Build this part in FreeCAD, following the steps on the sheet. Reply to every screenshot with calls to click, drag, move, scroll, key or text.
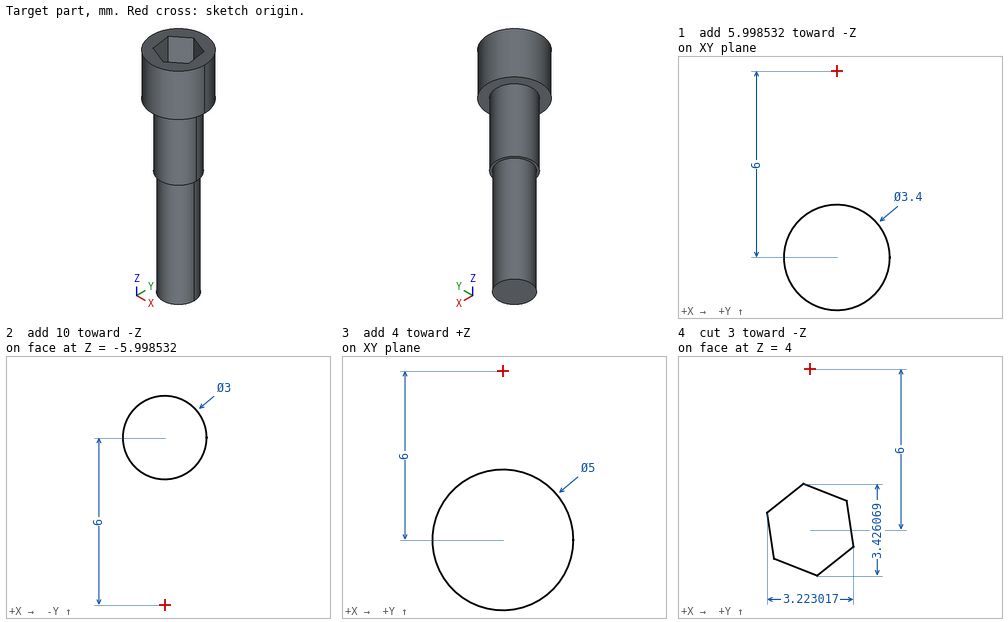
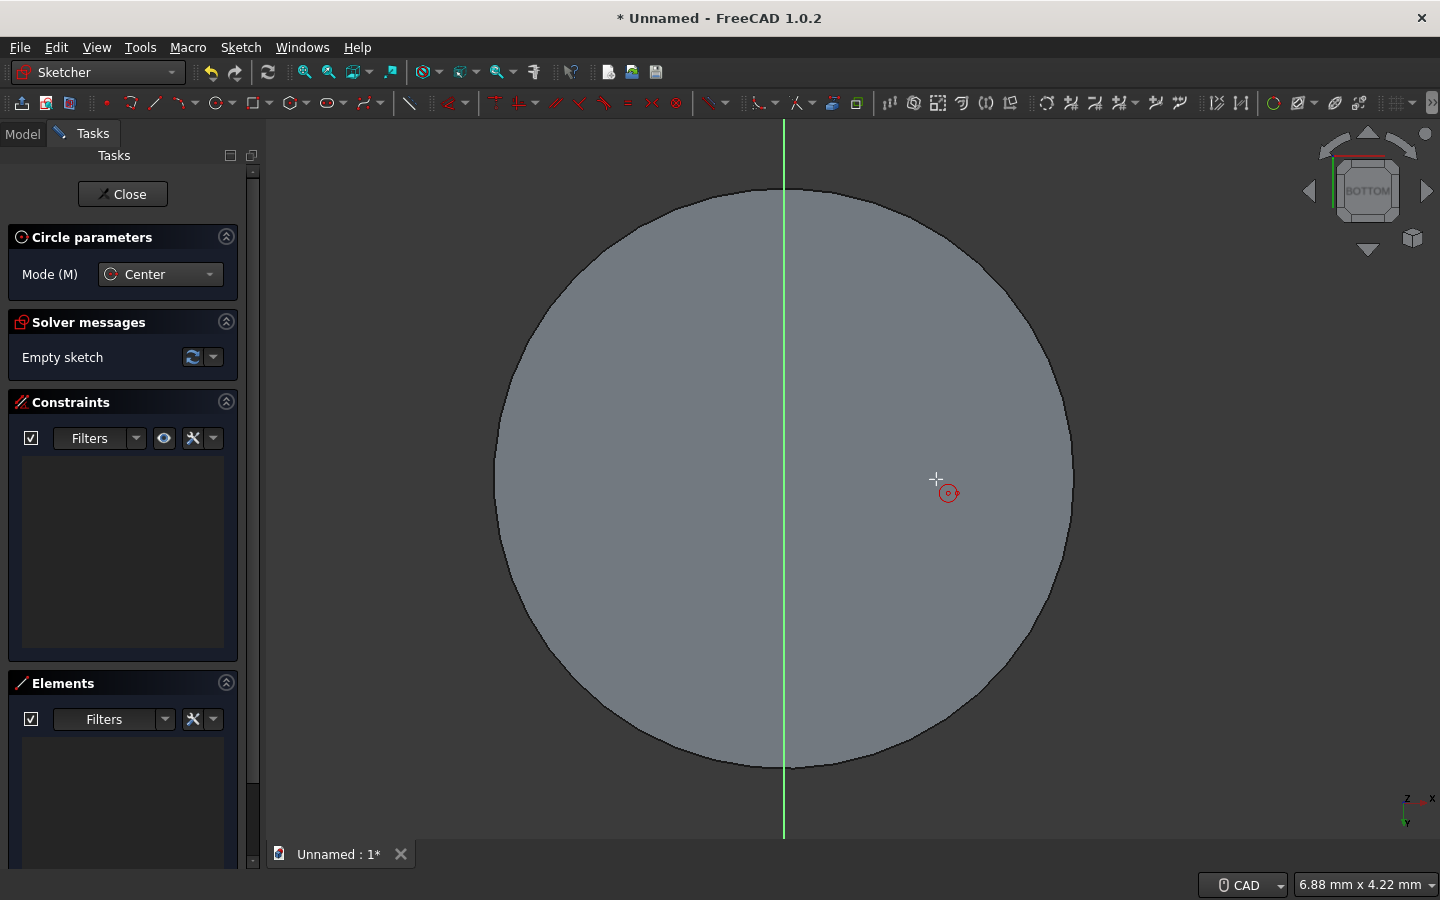
click(784, 479)
click(965, 298)
key(Escape)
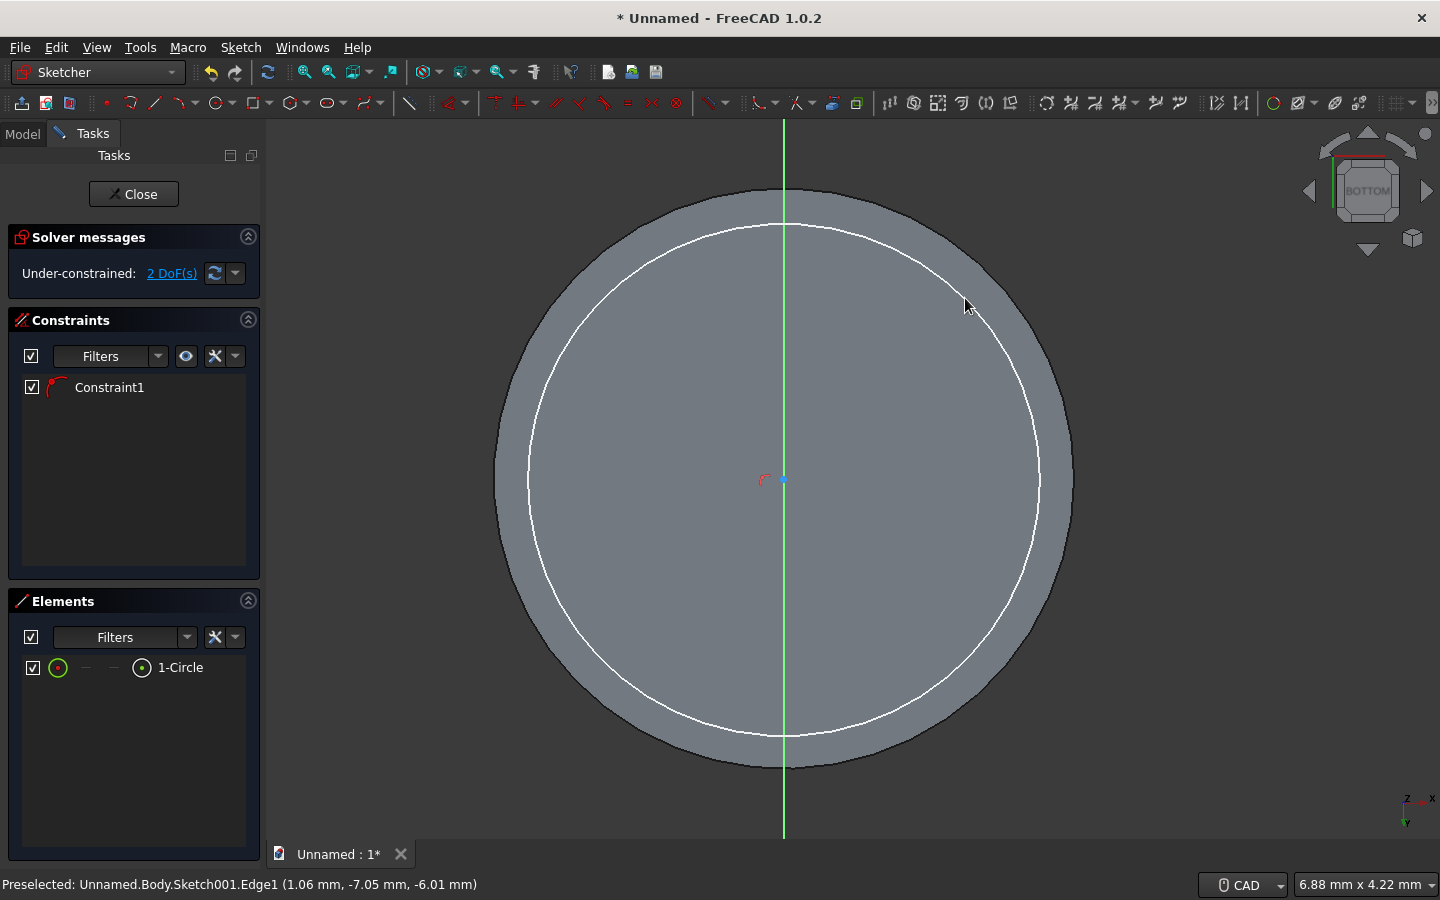
key(d)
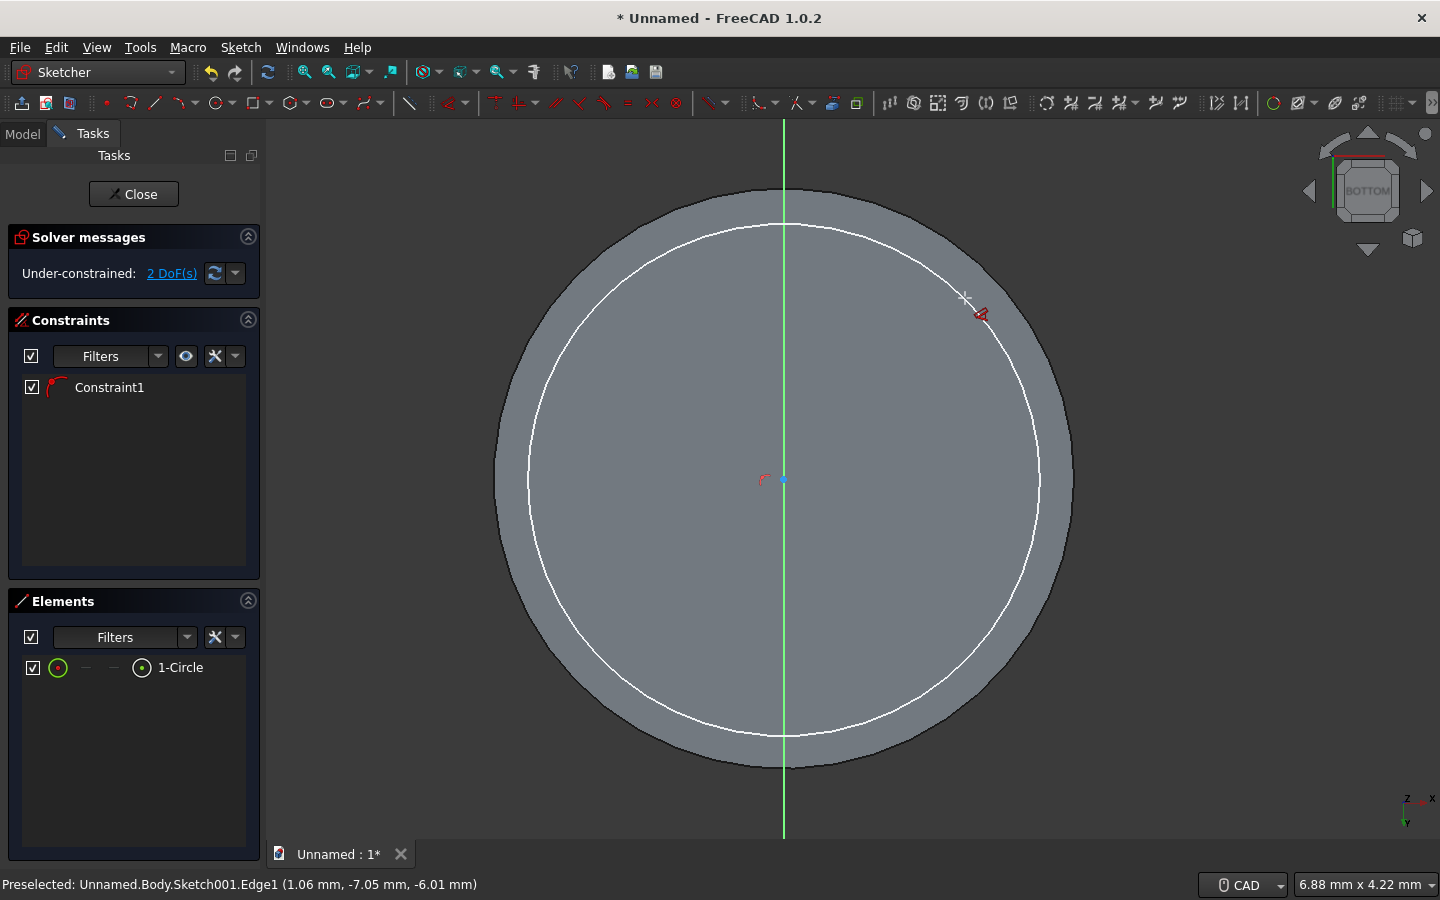
click(964, 298)
click(987, 275)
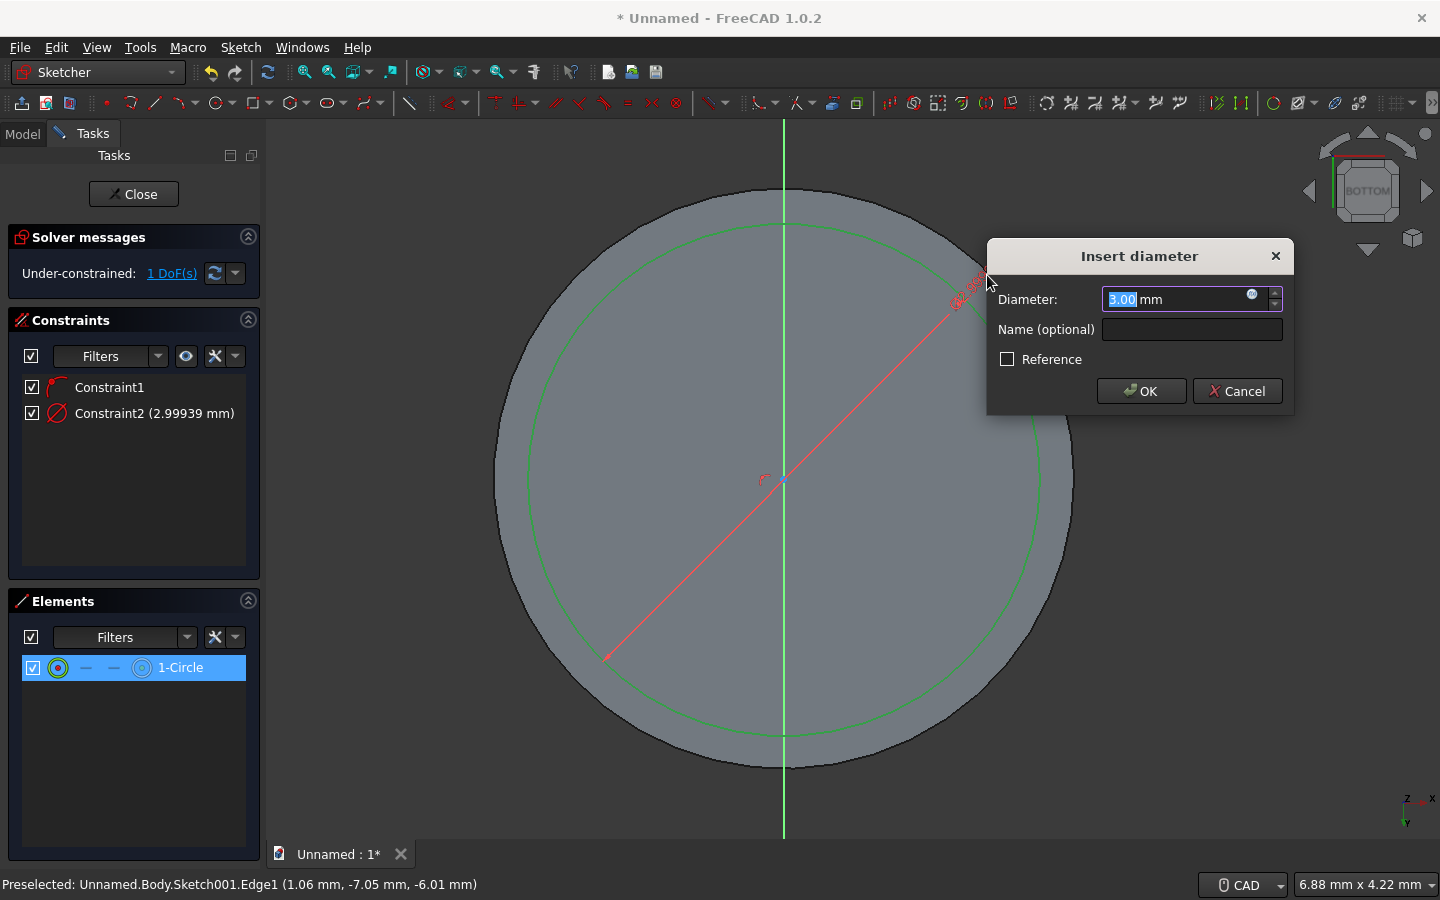
text(3)
key(Return)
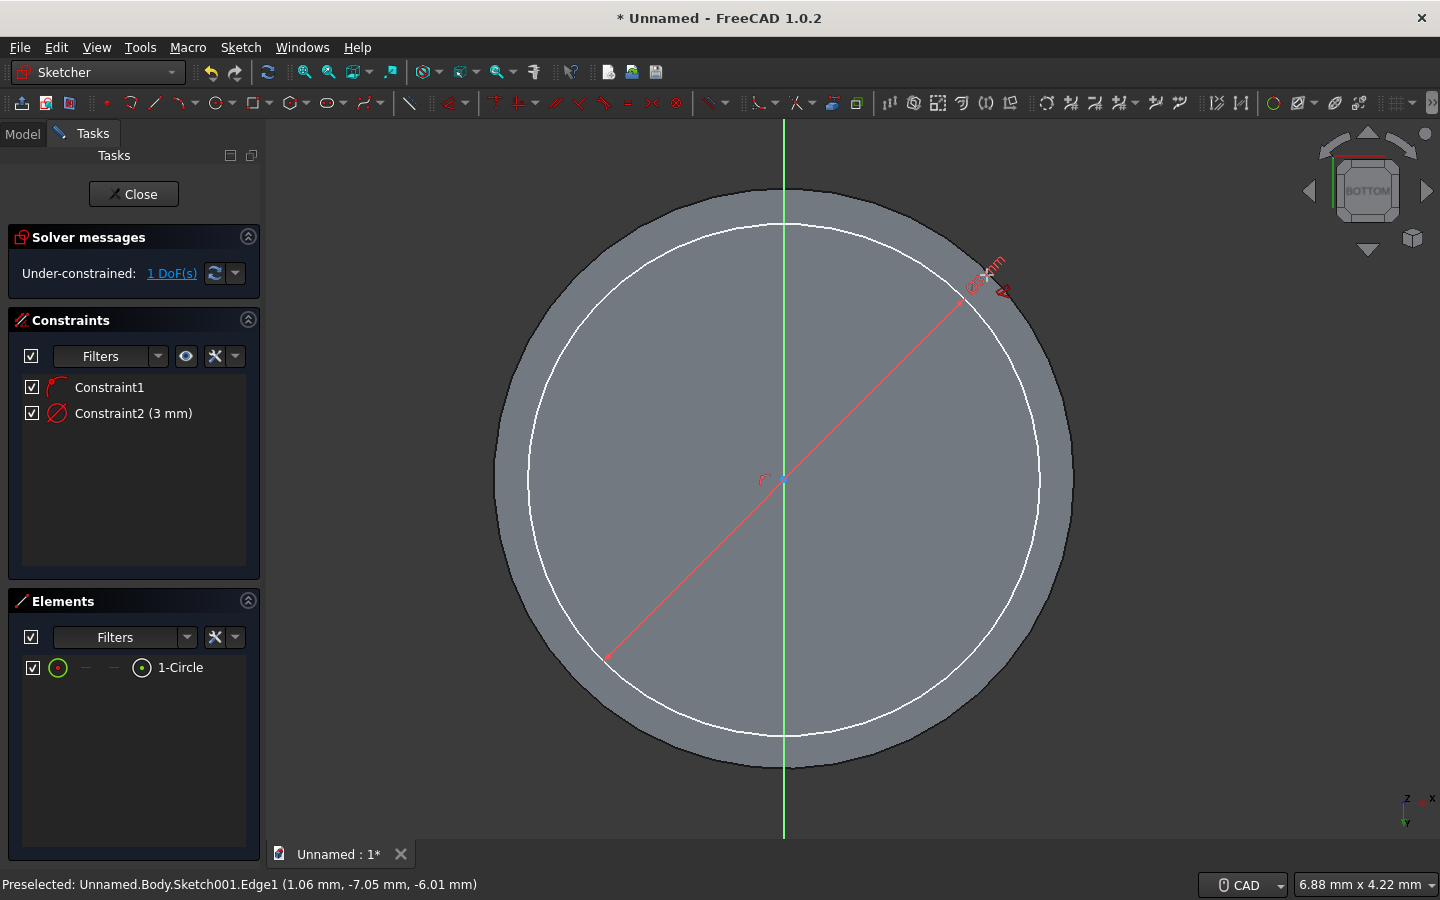
click(786, 482)
click(818, 645)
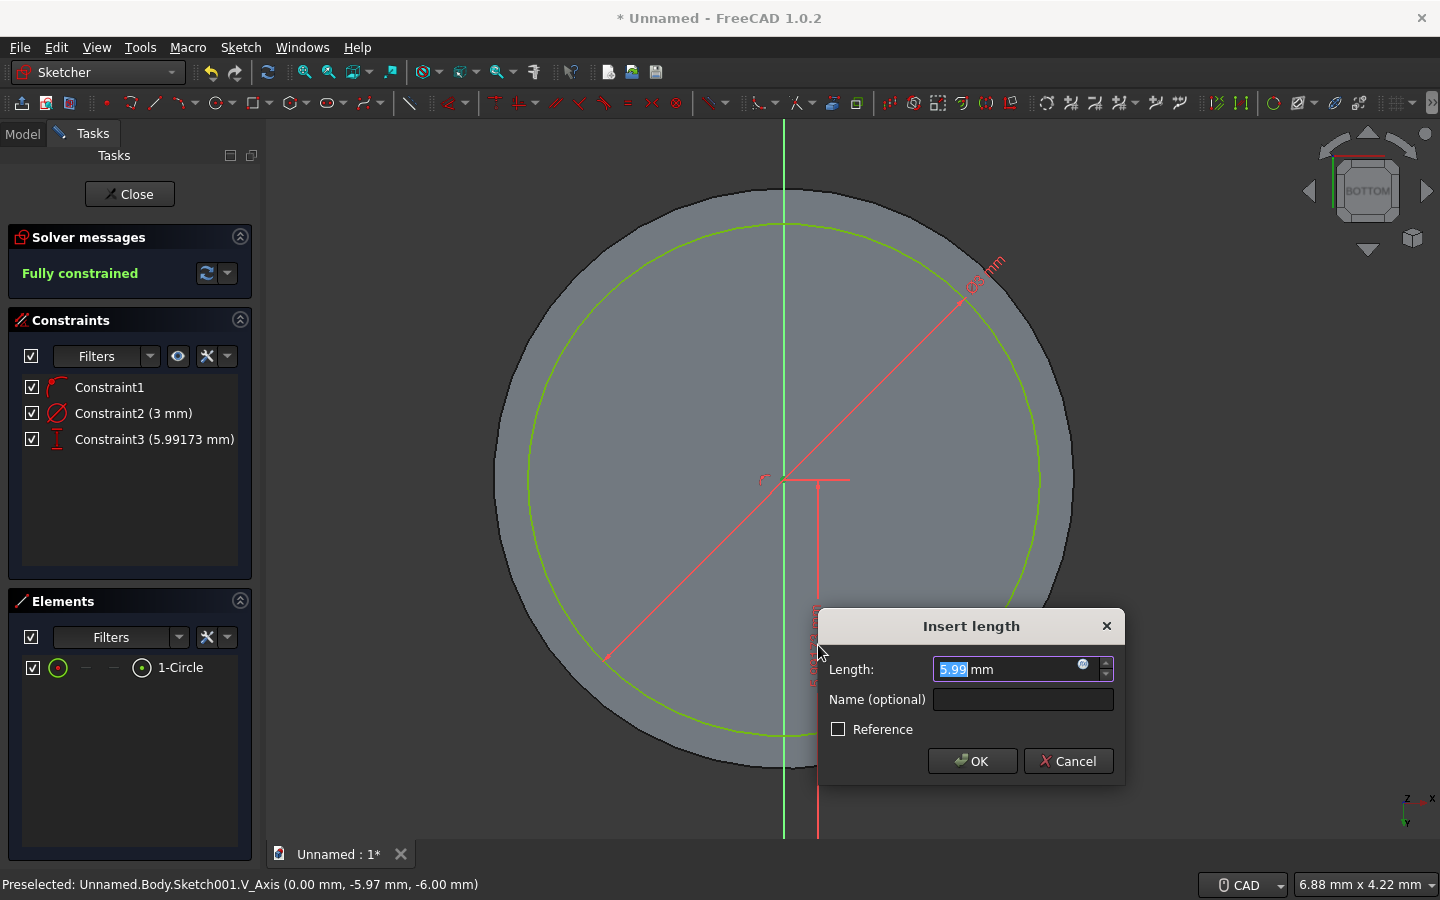
text(6)
key(Return)
key(Escape)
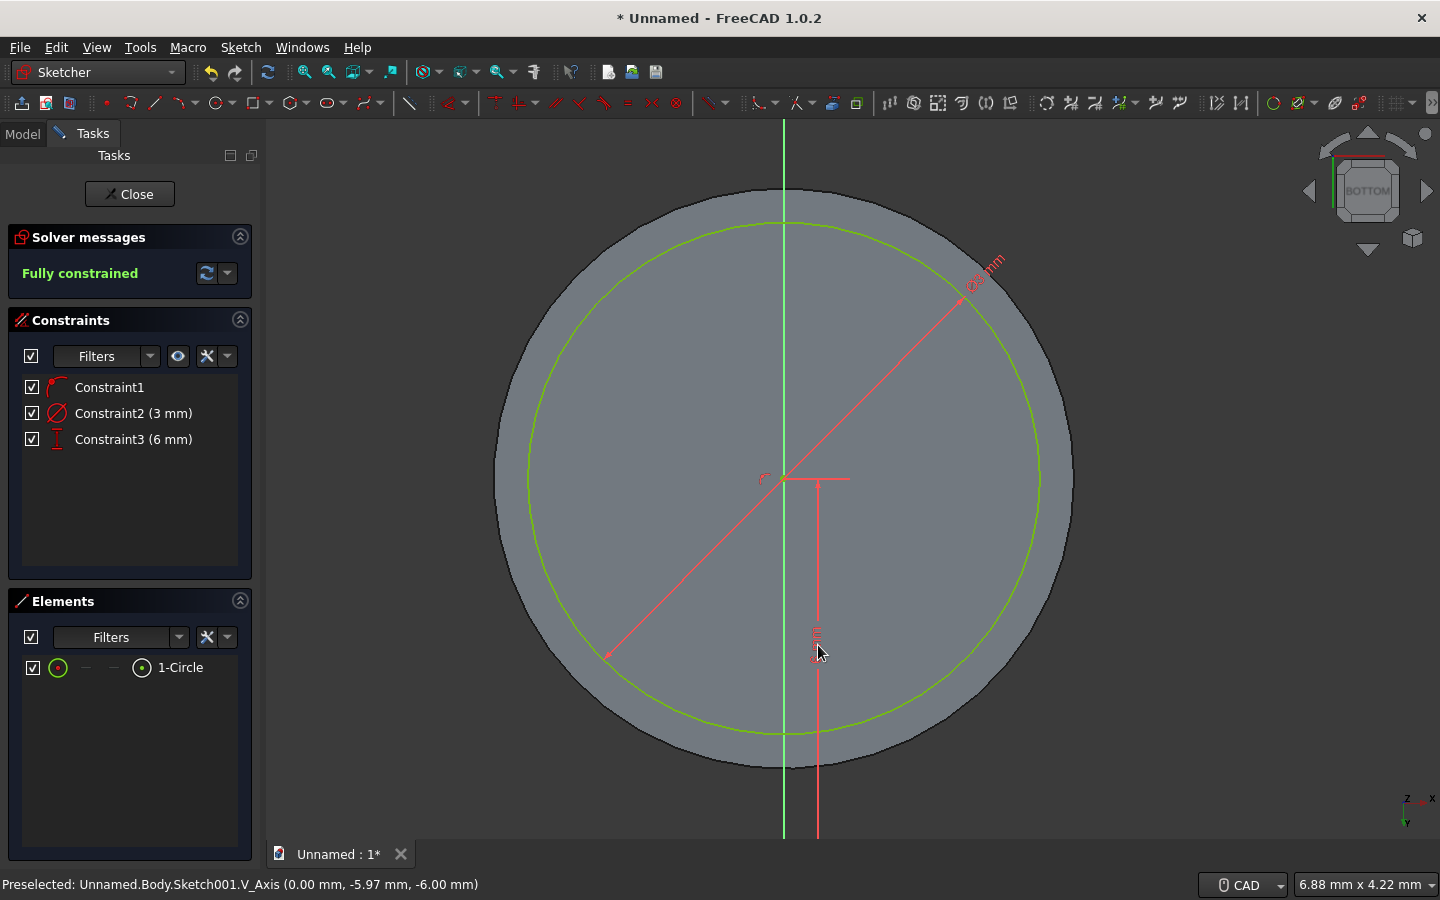
click(130, 194)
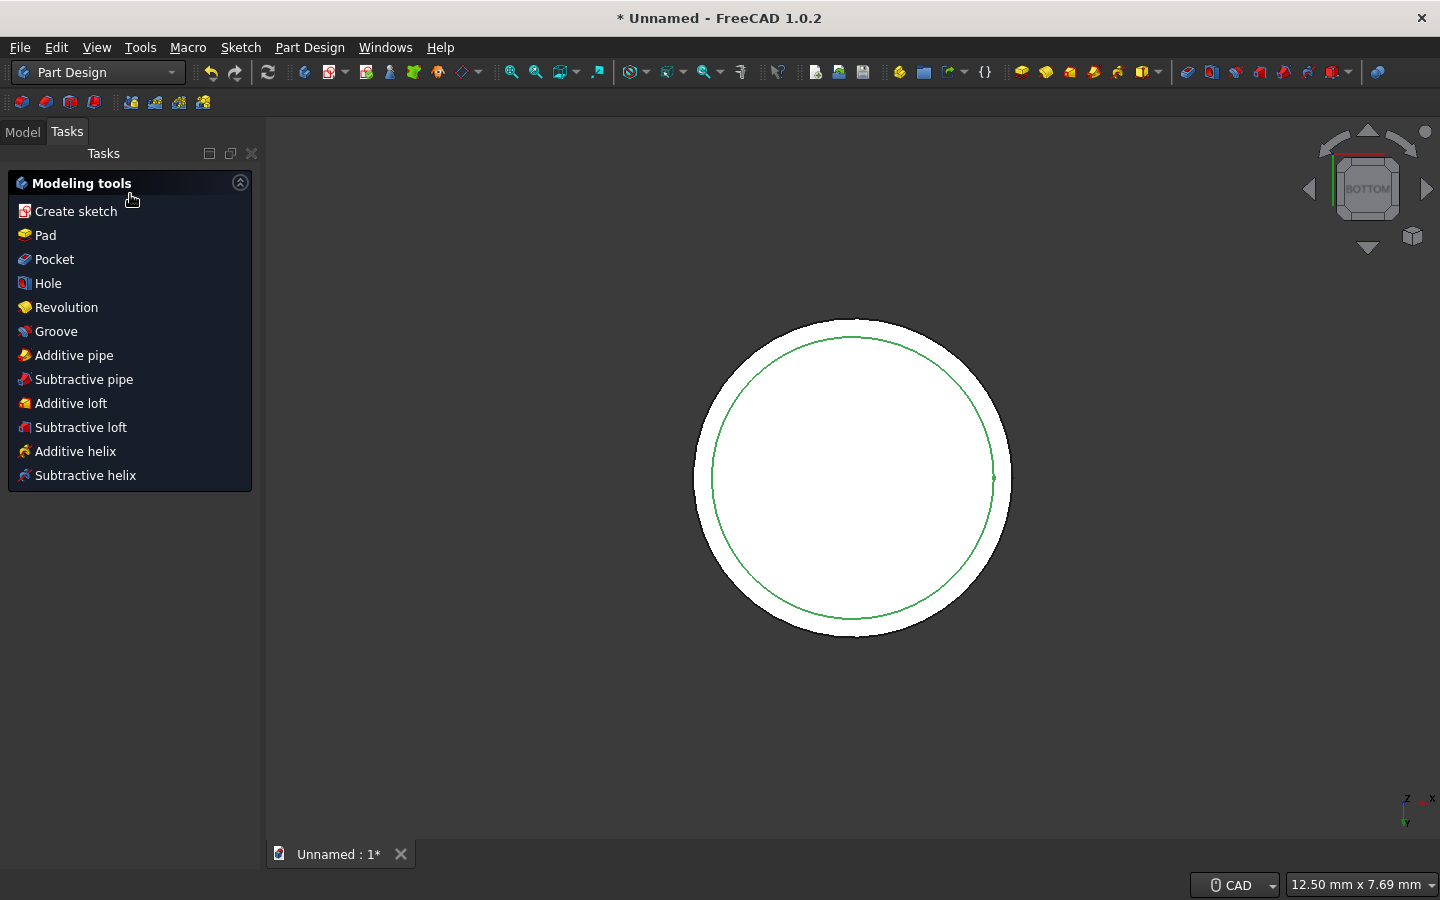
click(1022, 72)